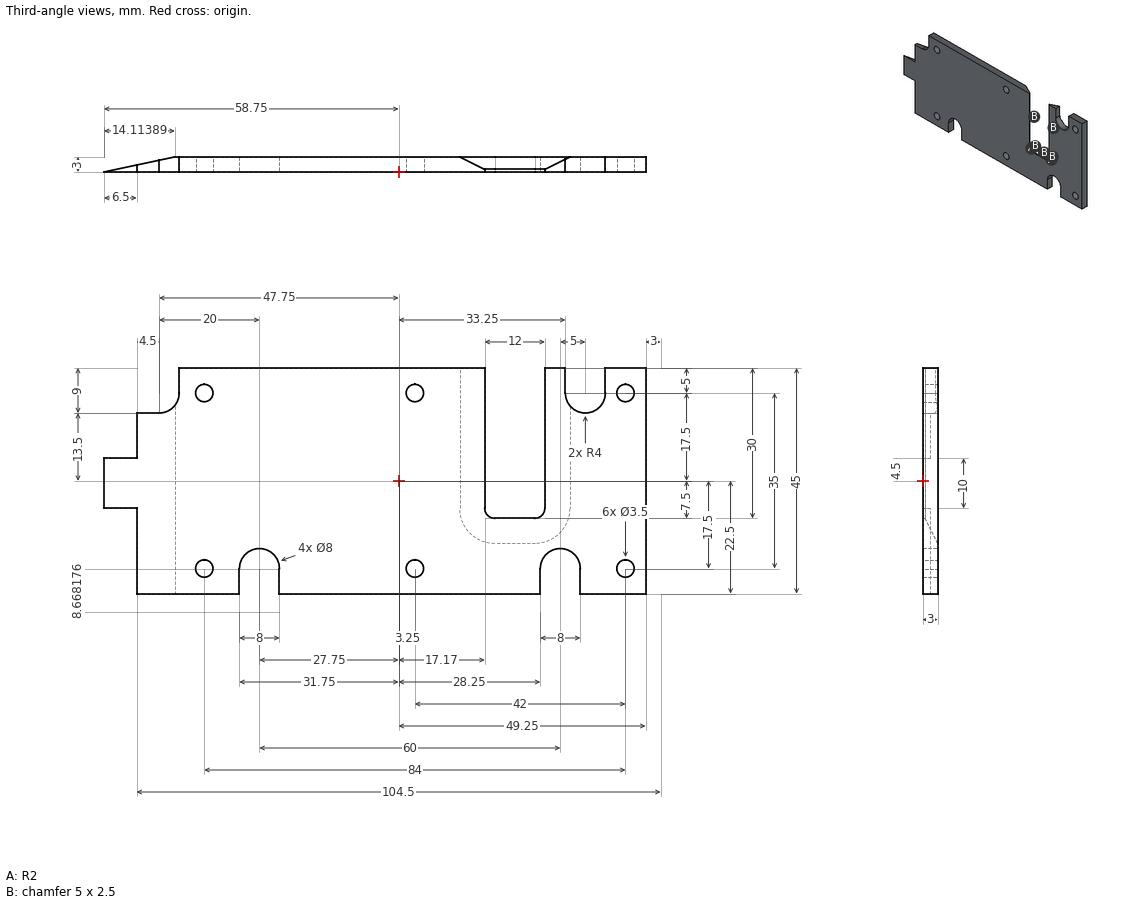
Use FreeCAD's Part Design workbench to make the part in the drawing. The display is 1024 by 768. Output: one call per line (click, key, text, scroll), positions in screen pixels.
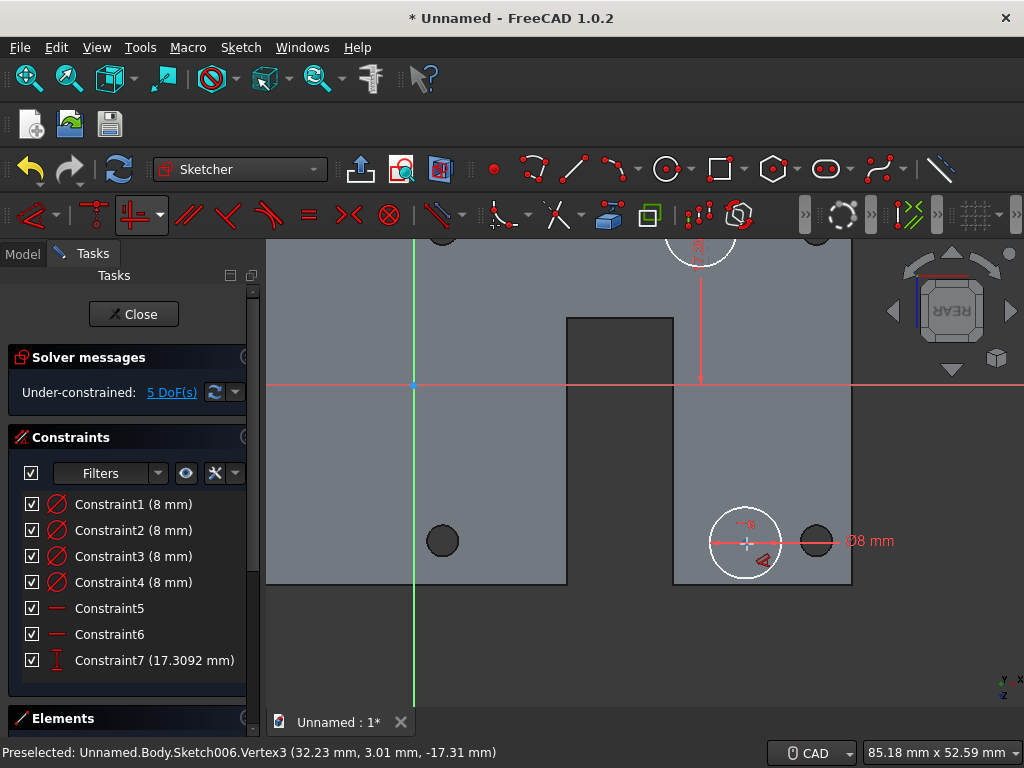
click(745, 543)
click(707, 577)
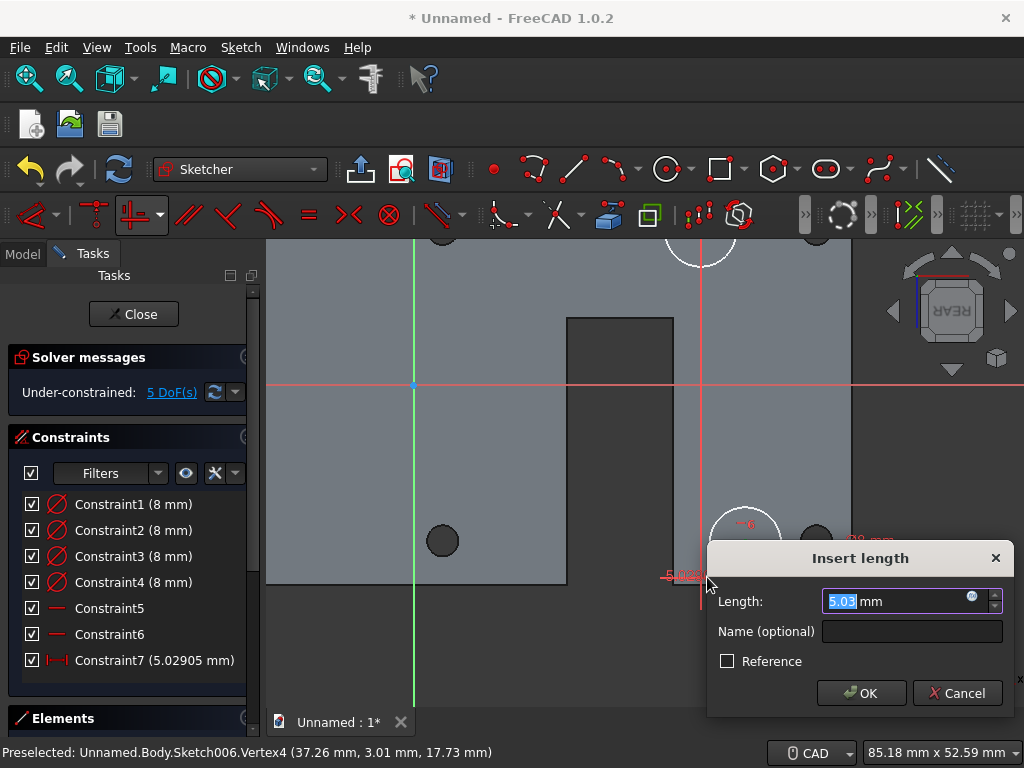
text(5)
key(Return)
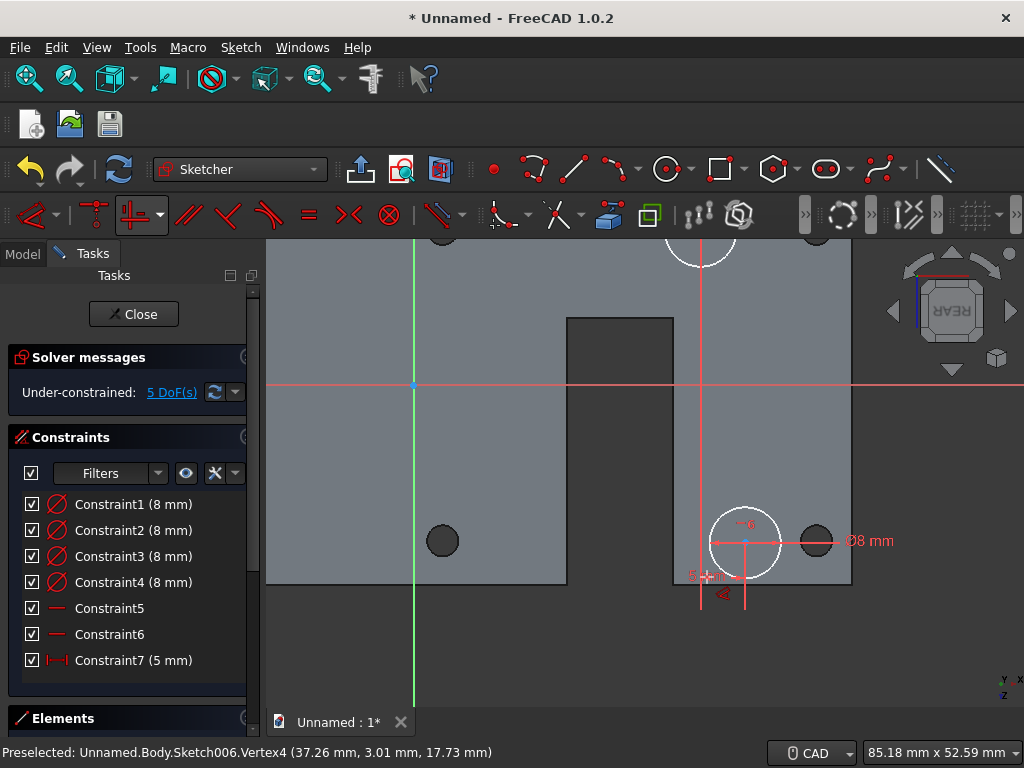
scroll(747, 545, down, 4)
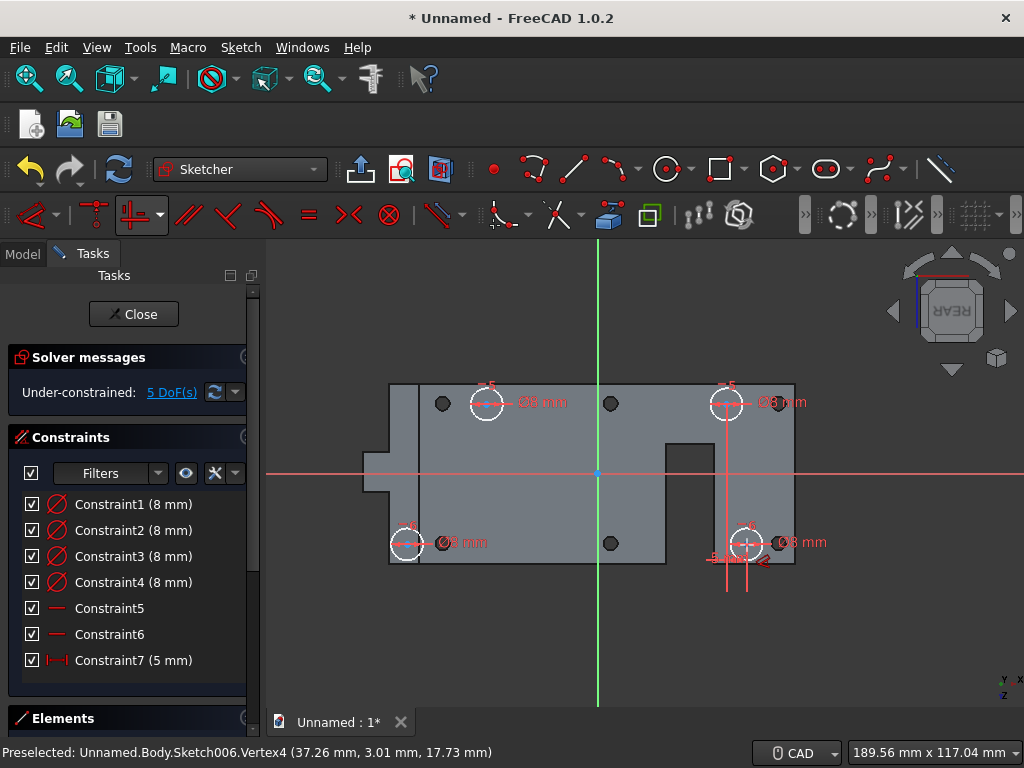
click(487, 404)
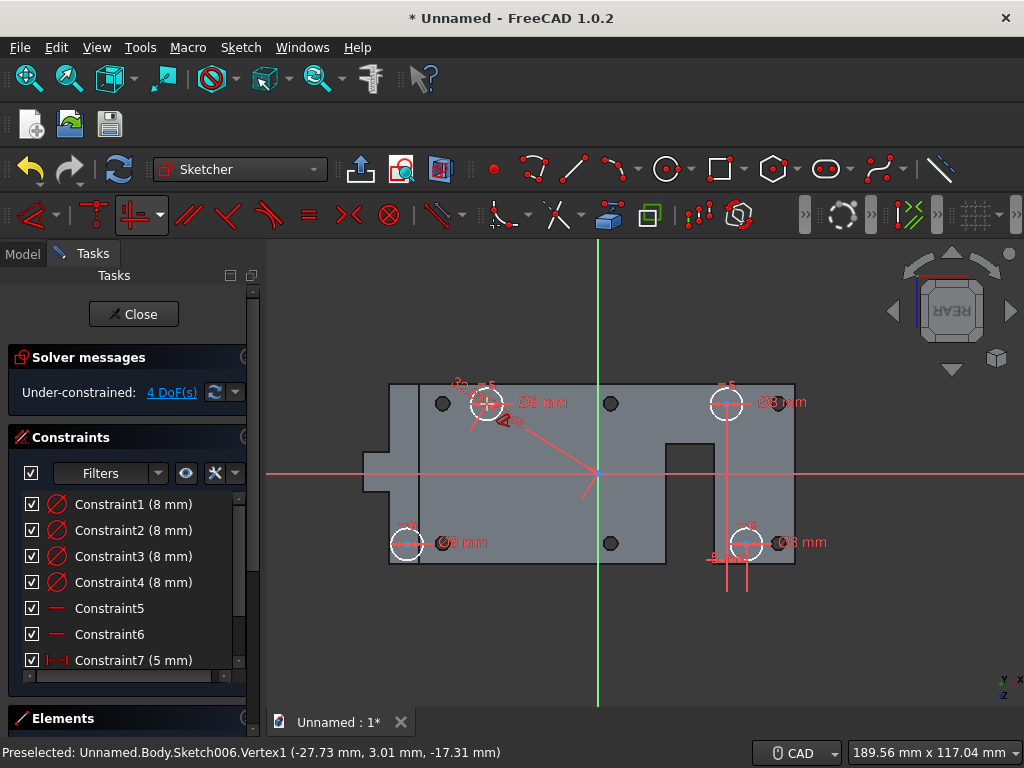
click(407, 544)
click(447, 578)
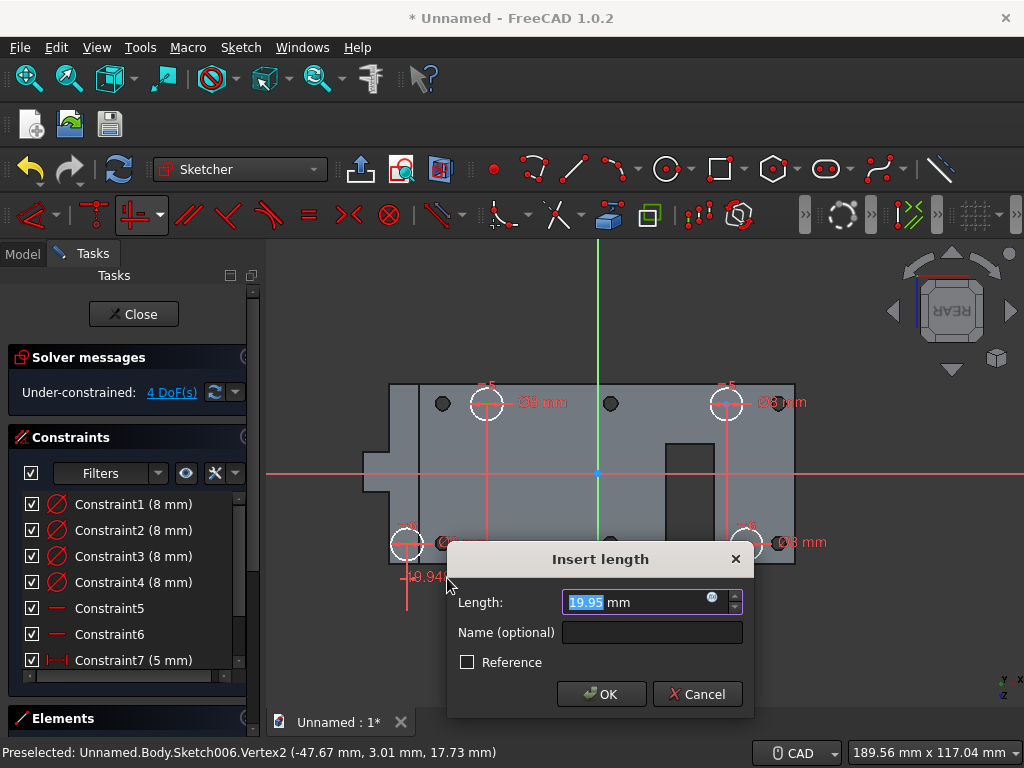
text(20)
key(Return)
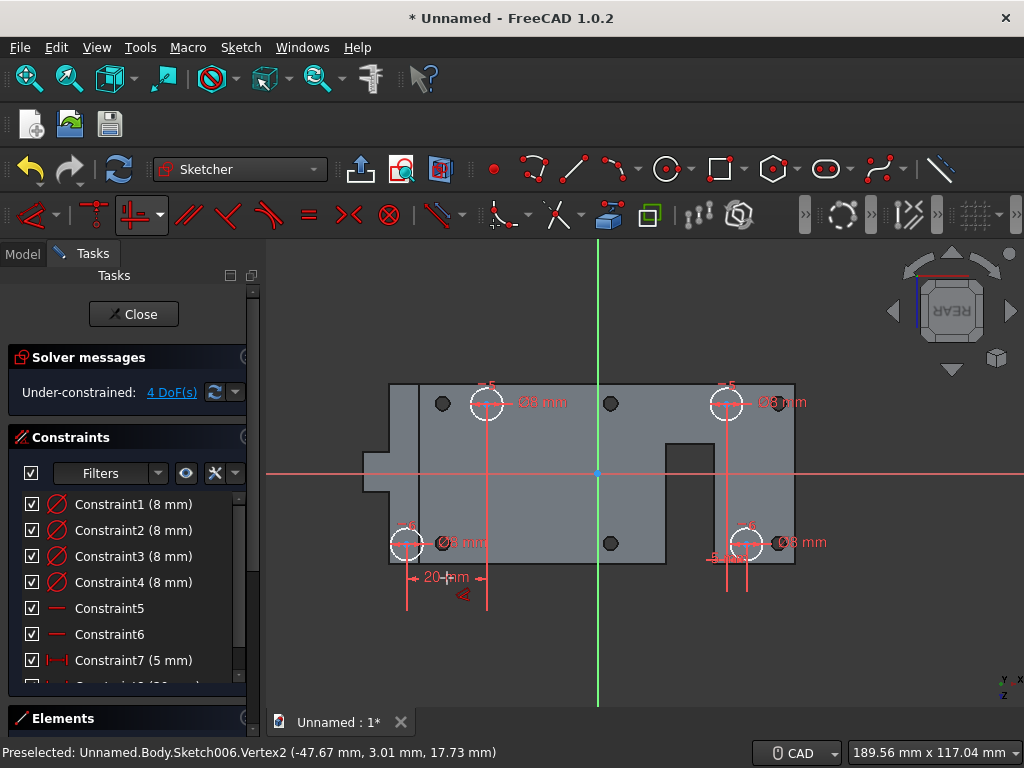
click(487, 404)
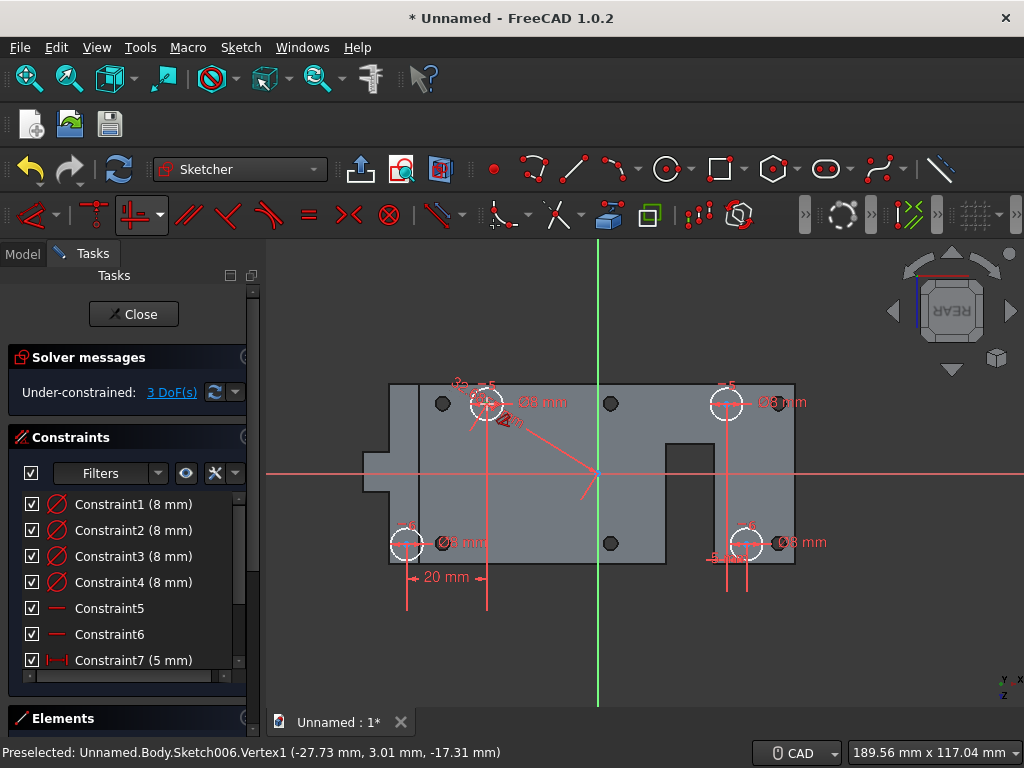
click(407, 544)
click(373, 442)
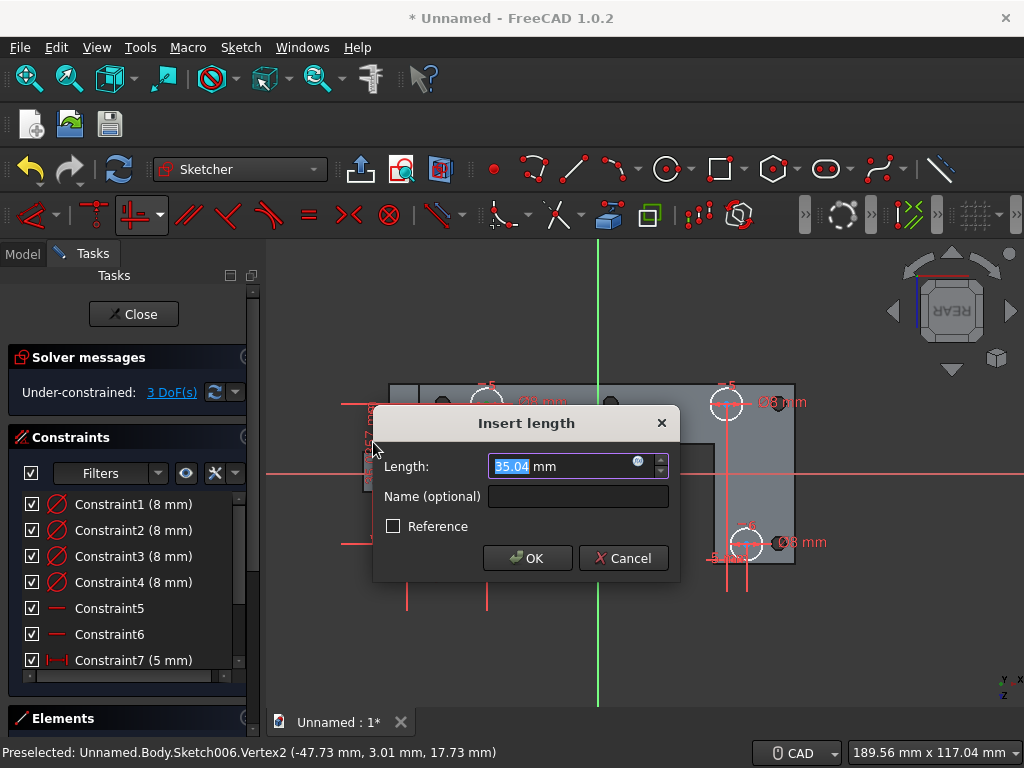
text(35)
key(Return)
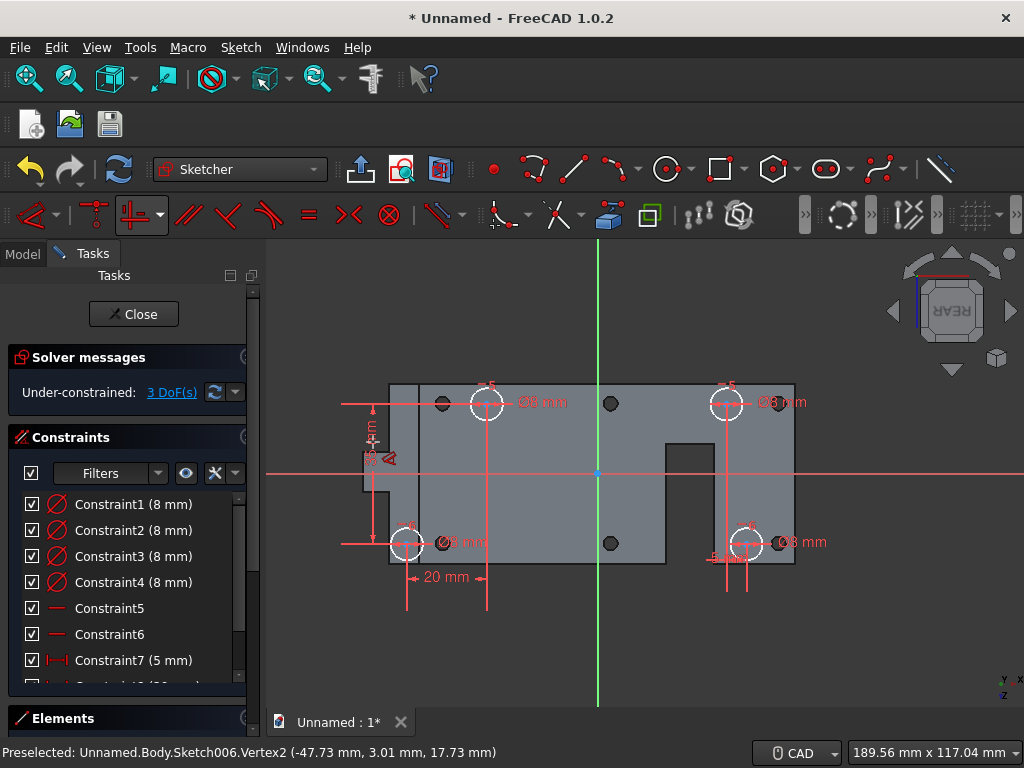
click(487, 404)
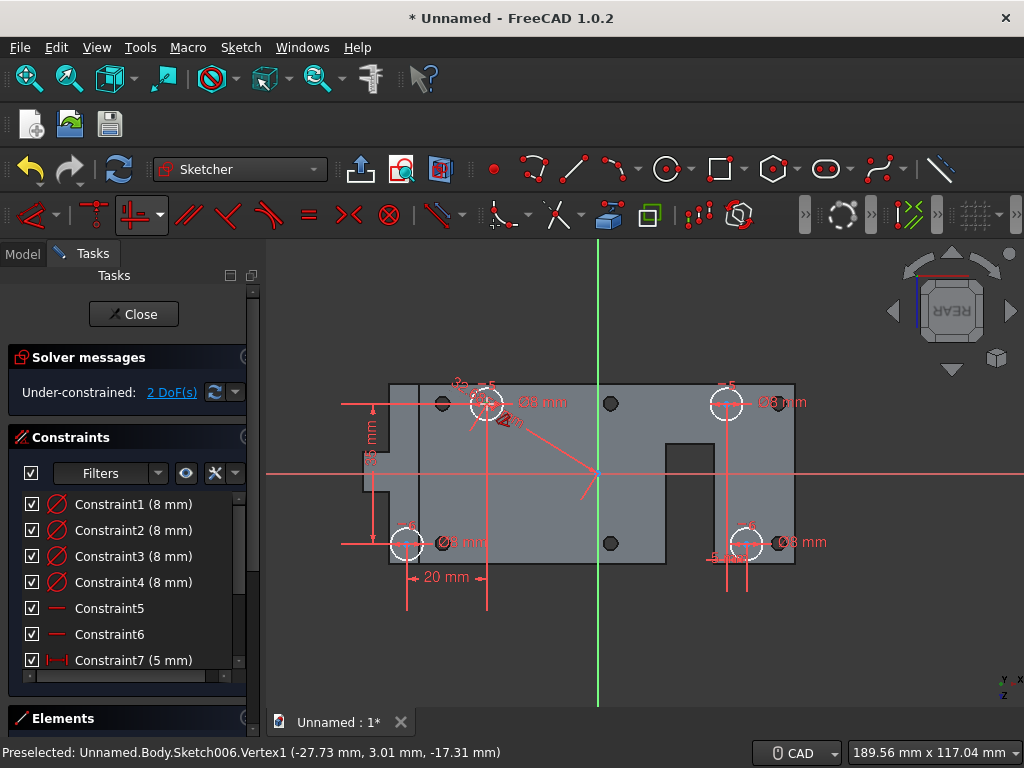
click(727, 404)
click(552, 370)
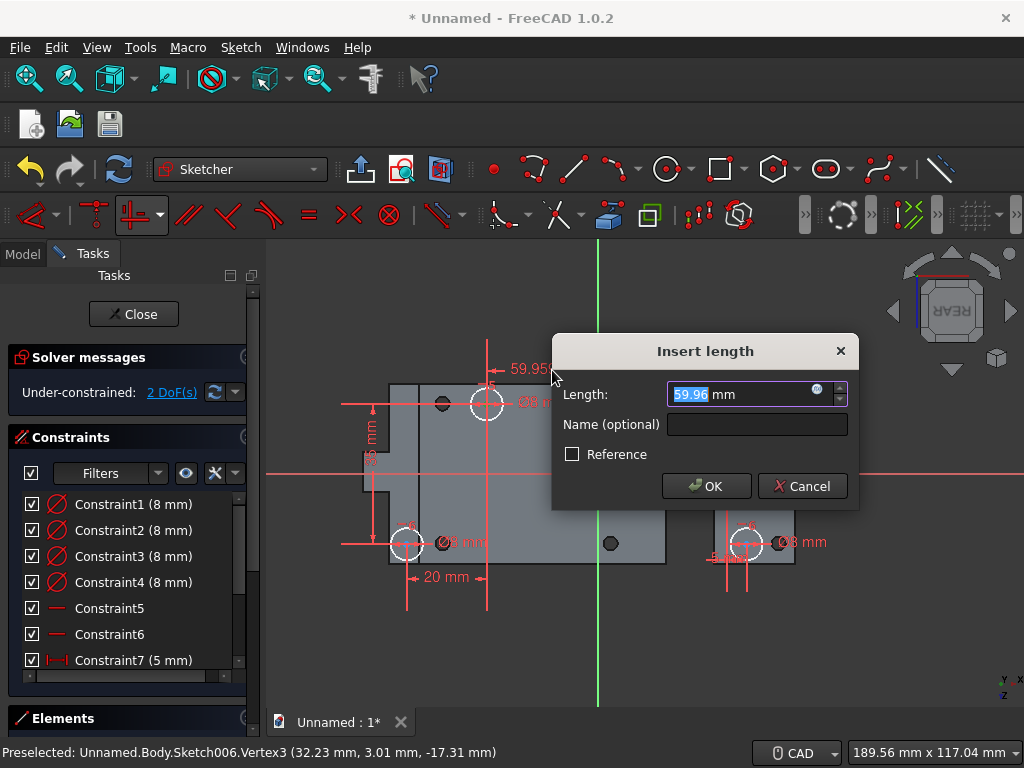
text(60)
key(Return)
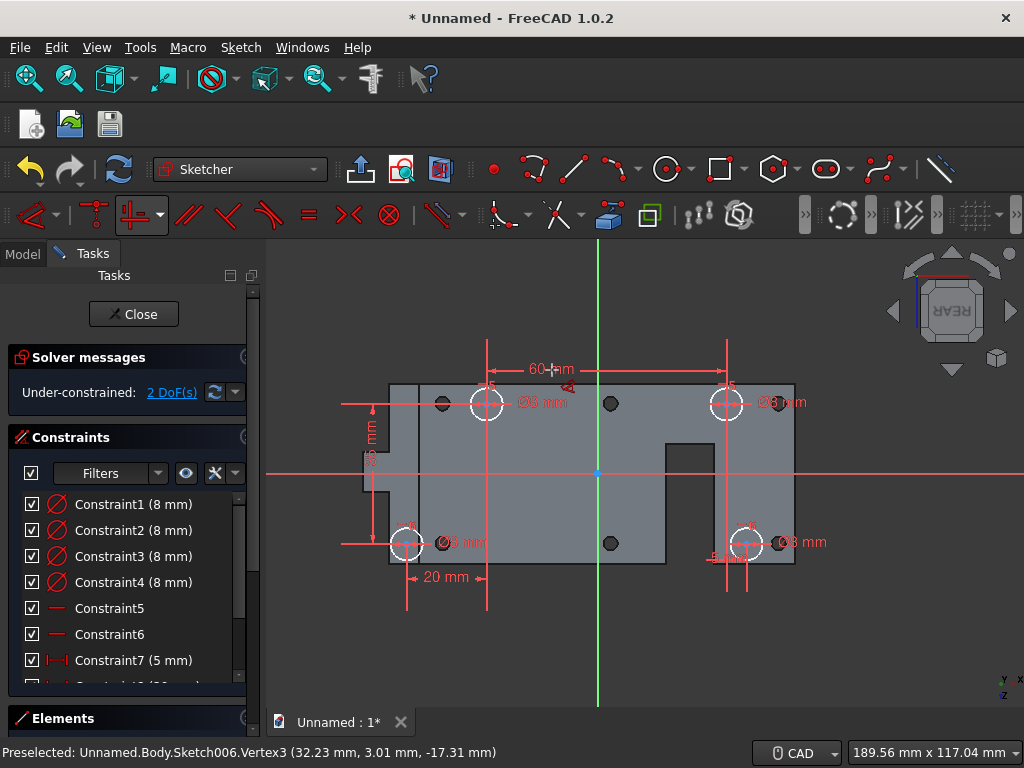
click(487, 404)
click(453, 439)